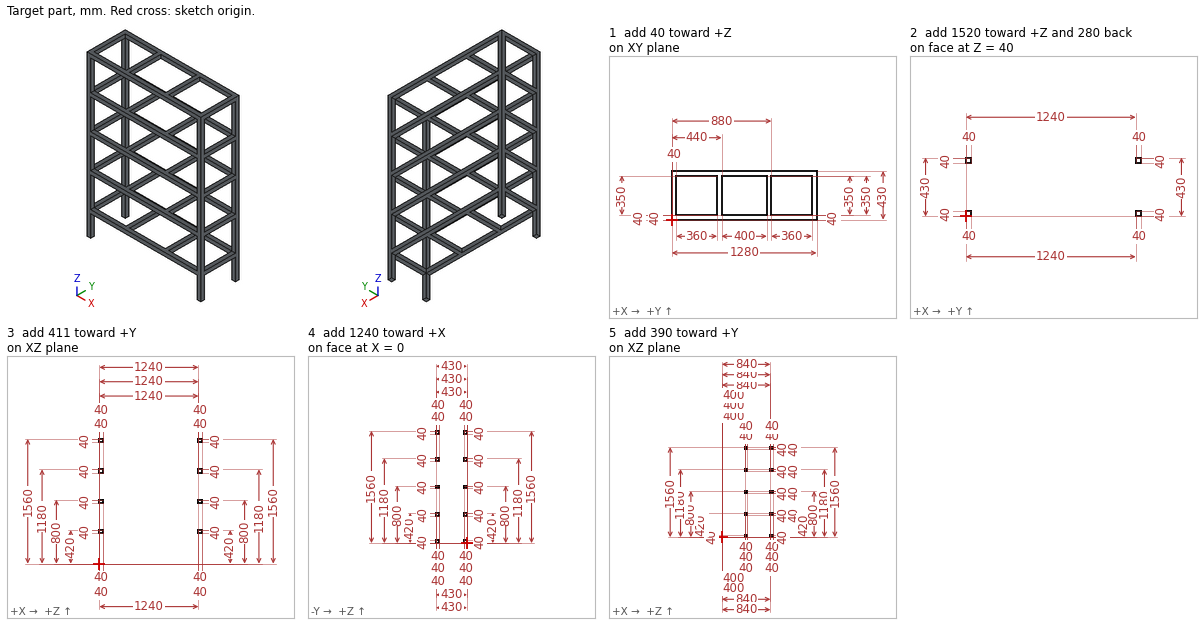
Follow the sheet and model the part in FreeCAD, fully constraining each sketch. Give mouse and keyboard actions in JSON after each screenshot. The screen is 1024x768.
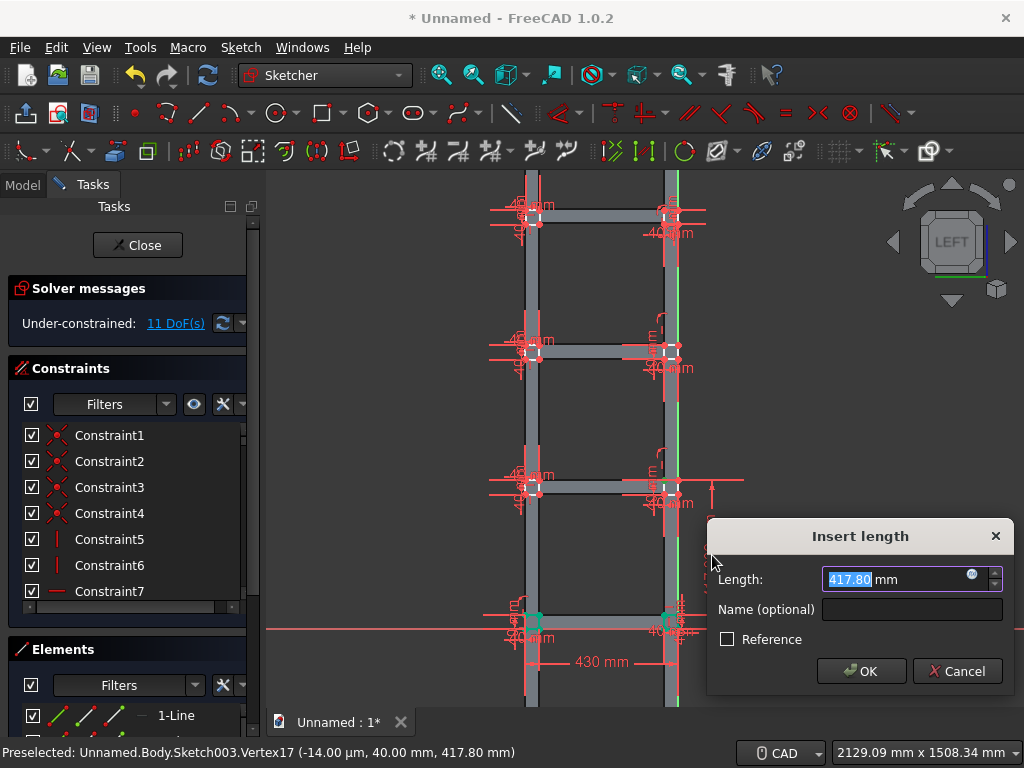
{"action": "type", "text": "420"}
{"action": "key", "text": "Return"}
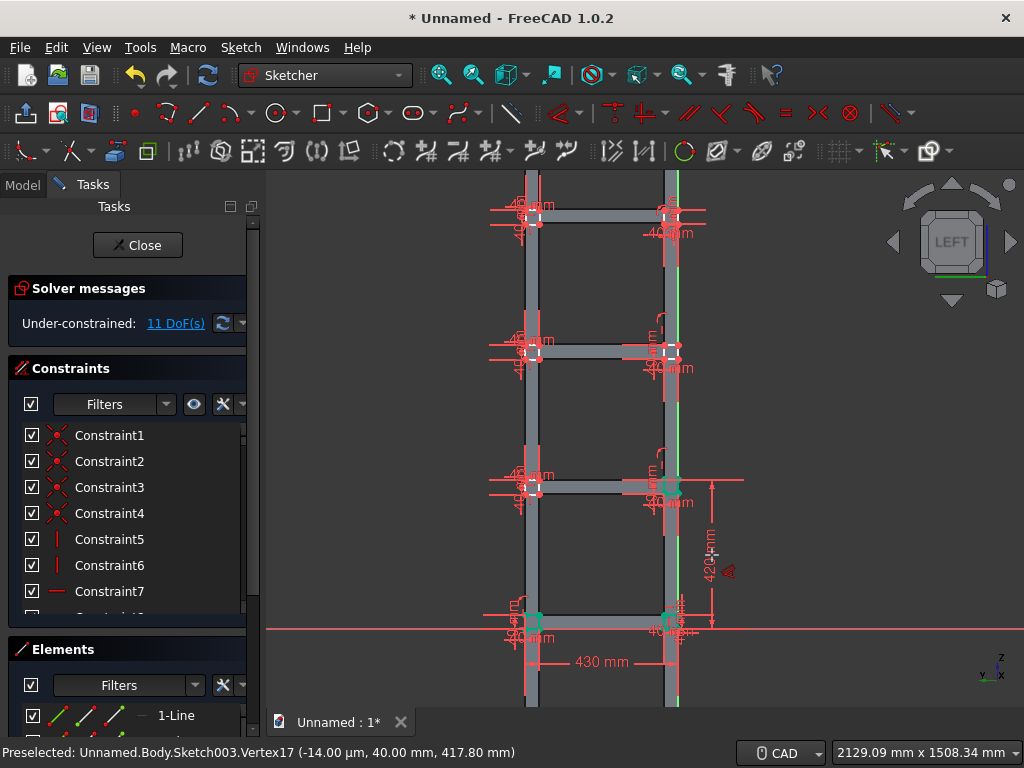
{"action": "left_click", "coordinate": [525, 480]}
{"action": "left_click", "coordinate": [602, 446]}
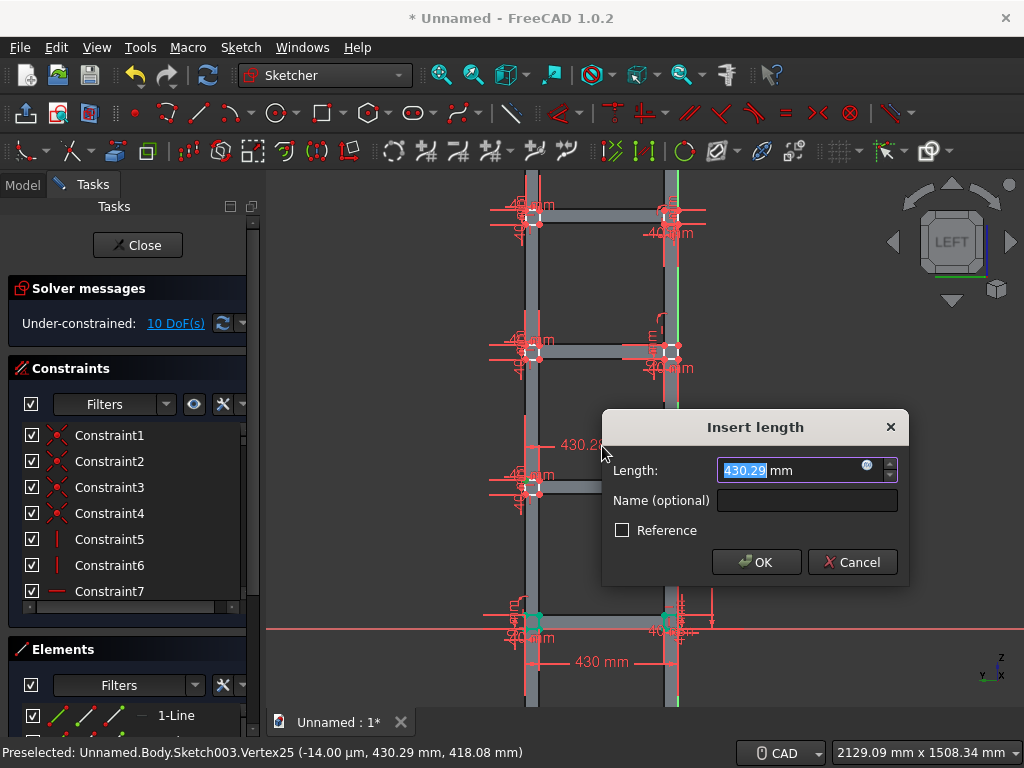
{"action": "type", "text": "430"}
{"action": "key", "text": "Return"}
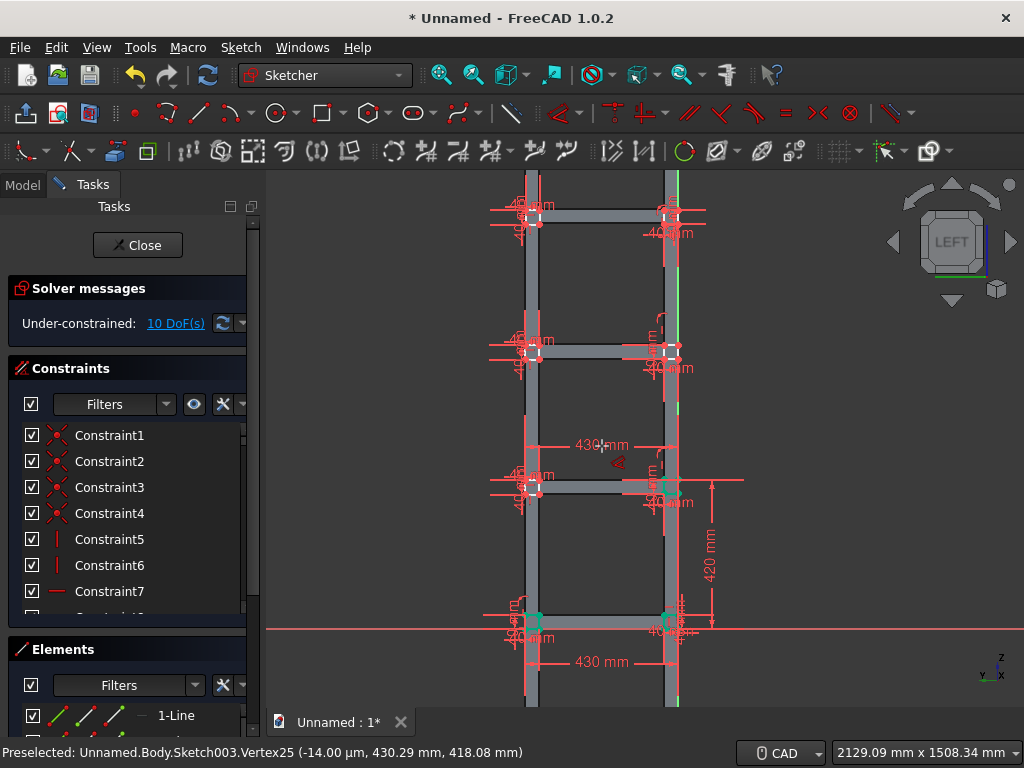
{"action": "left_click", "coordinate": [525, 480]}
{"action": "left_click", "coordinate": [712, 589]}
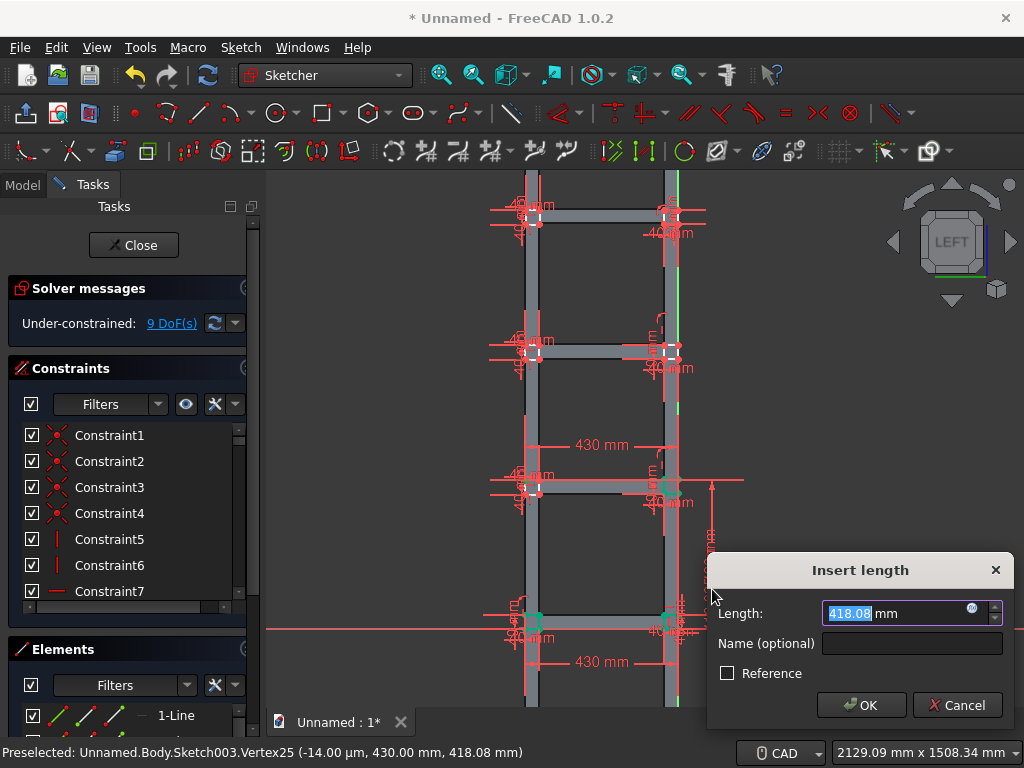
{"action": "type", "text": "420"}
{"action": "key", "text": "Return"}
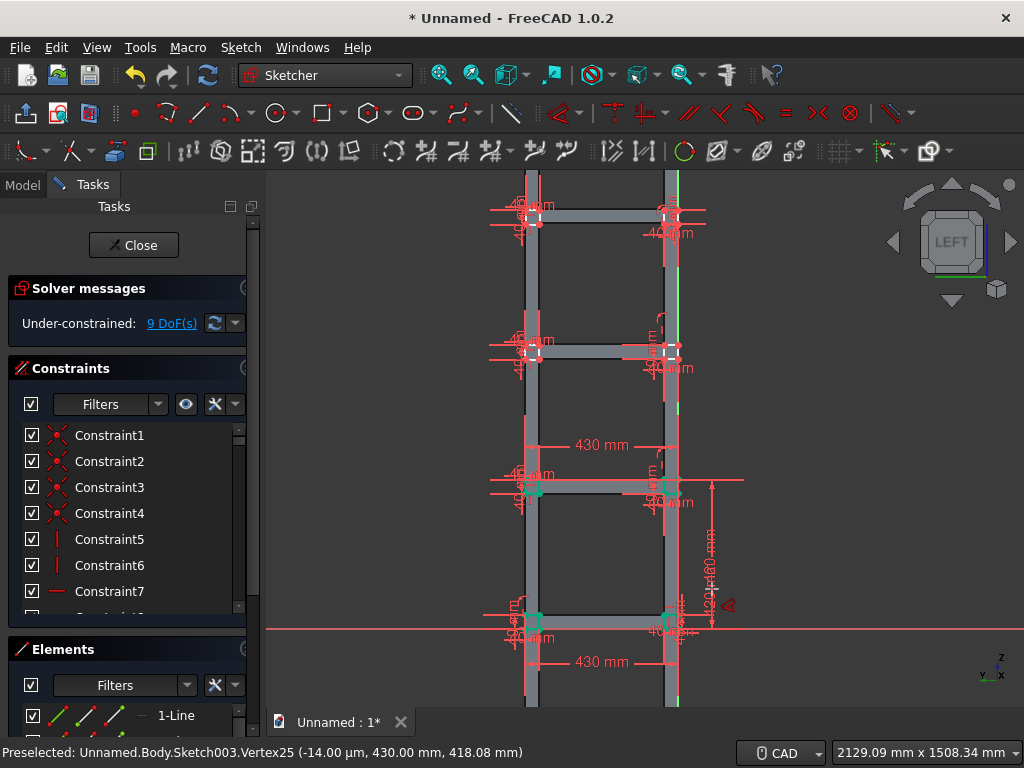
{"action": "left_click", "coordinate": [525, 345]}
{"action": "left_click", "coordinate": [602, 311]}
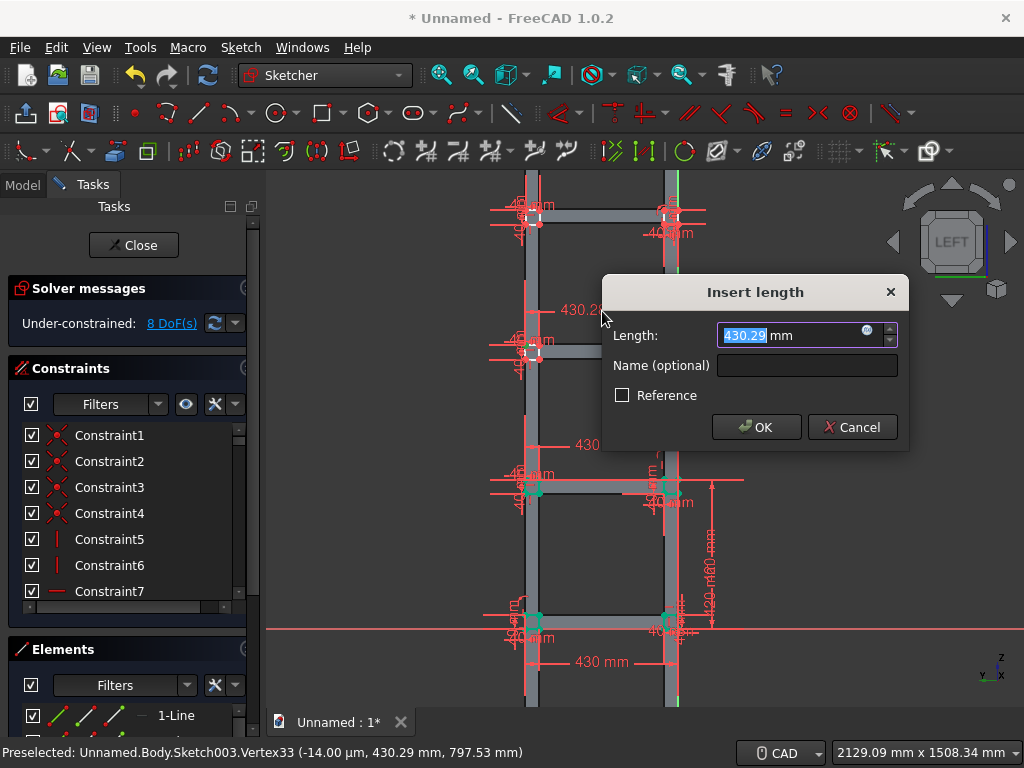
{"action": "type", "text": "430"}
{"action": "key", "text": "Return"}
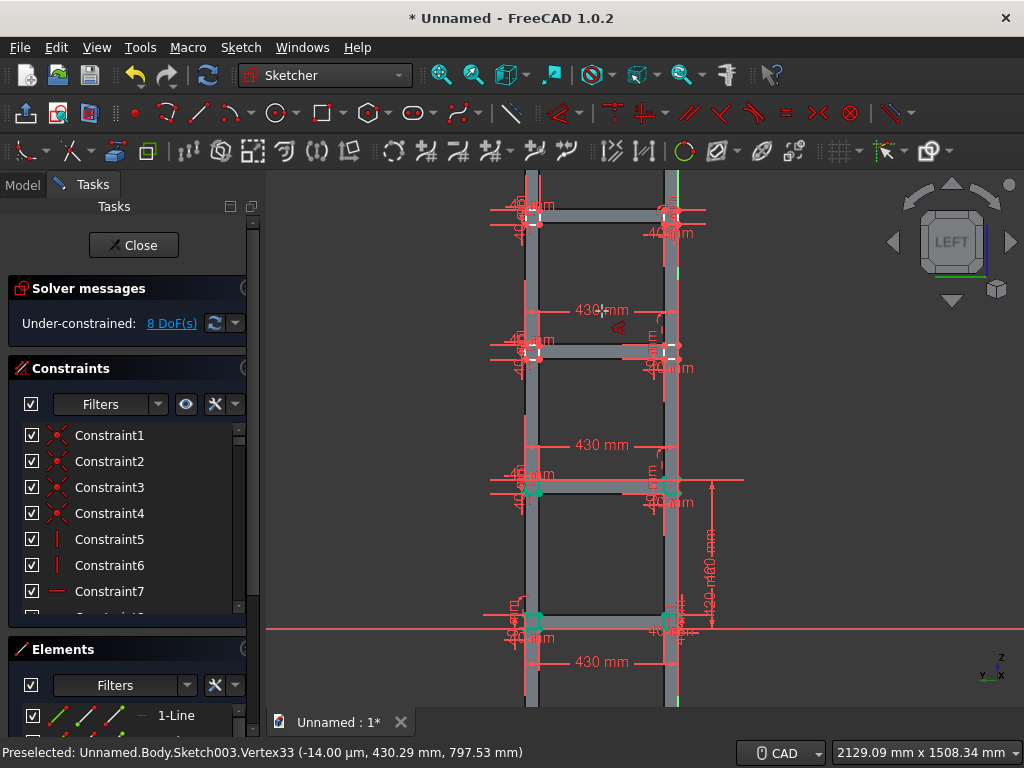
{"action": "left_click", "coordinate": [525, 345]}
{"action": "left_click", "coordinate": [712, 422]}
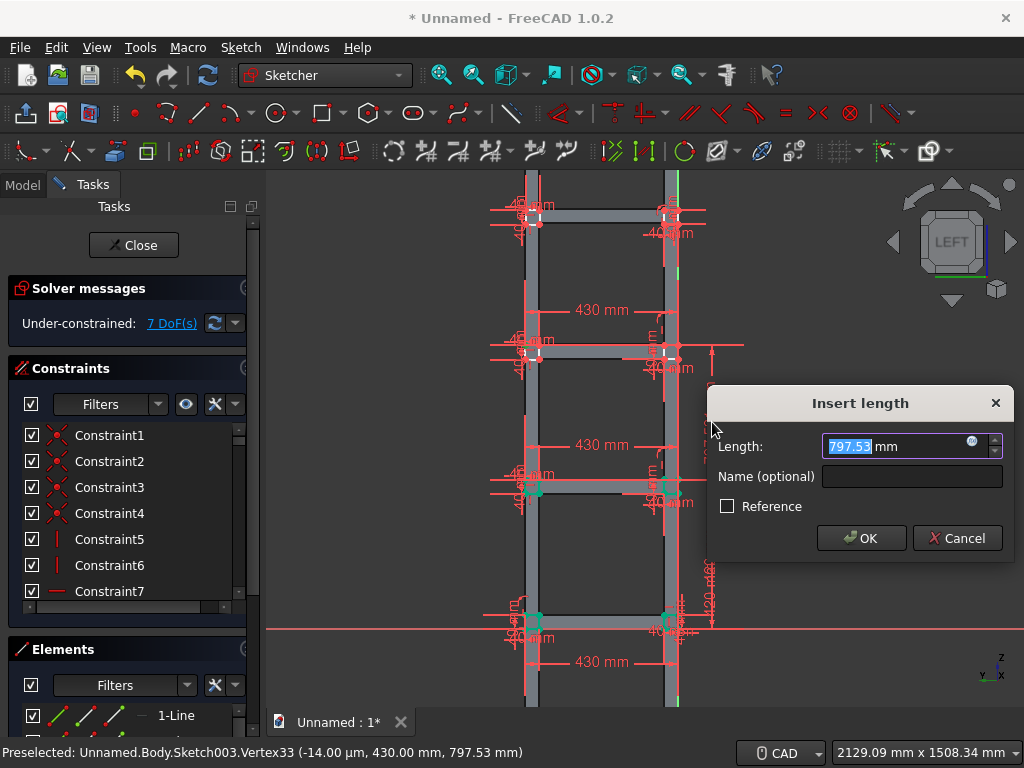
{"action": "type", "text": "800"}
{"action": "key", "text": "Return"}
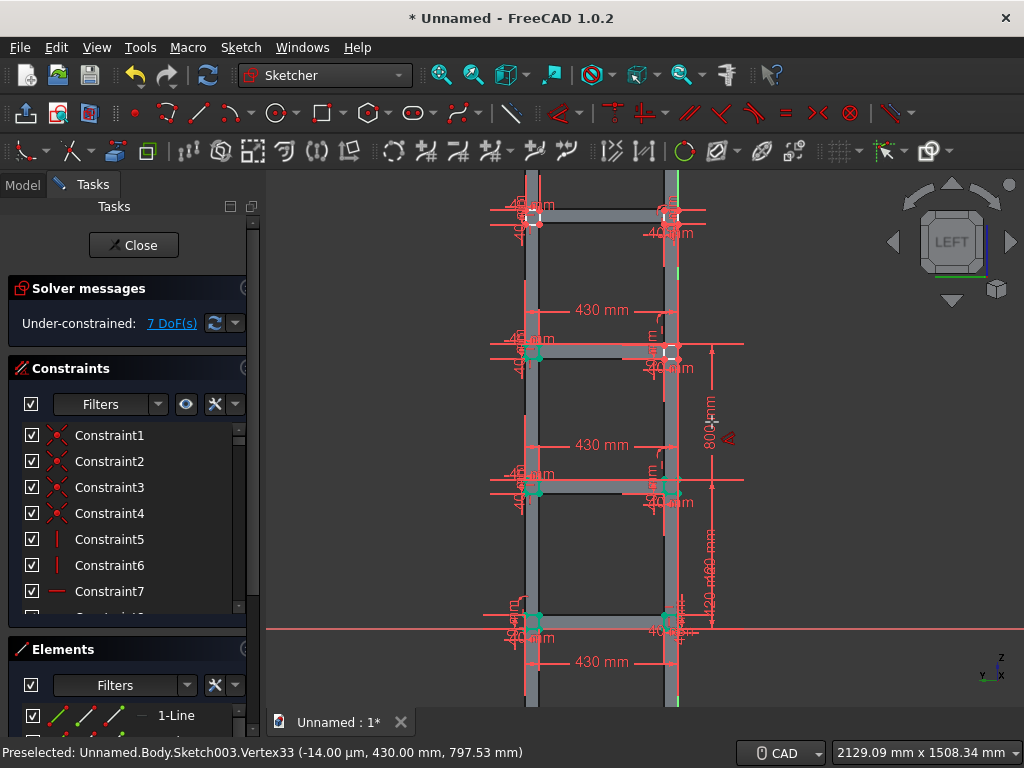
{"action": "left_click", "coordinate": [664, 345]}
{"action": "left_click", "coordinate": [630, 422]}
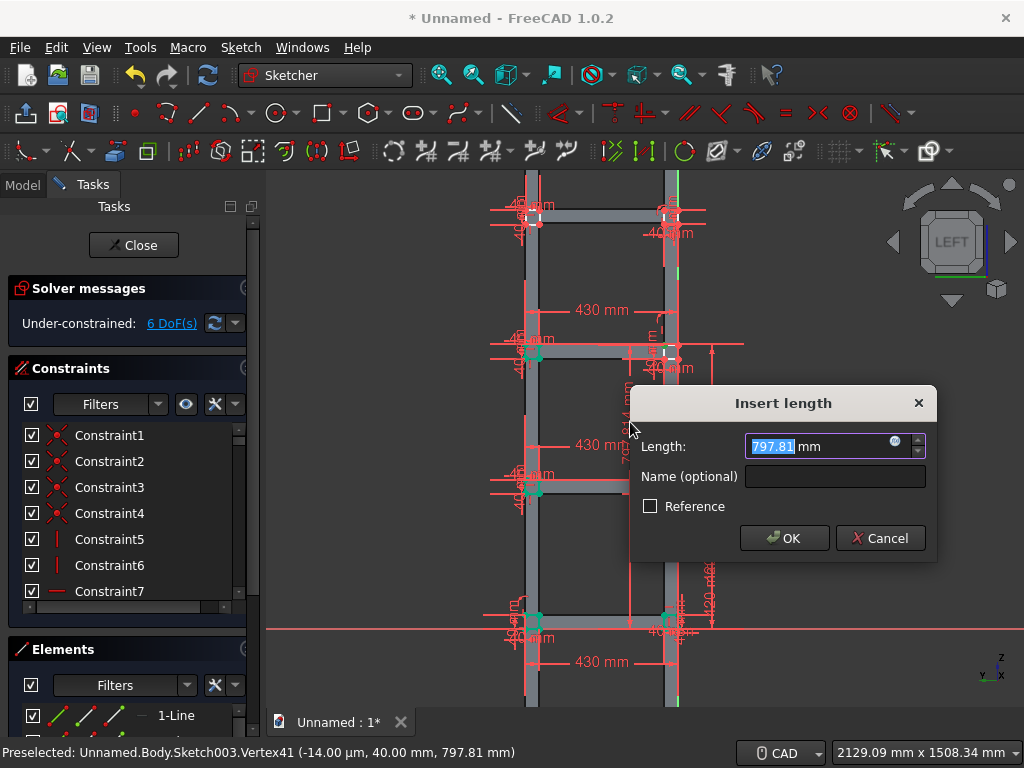
{"action": "type", "text": "800"}
{"action": "key", "text": "Return"}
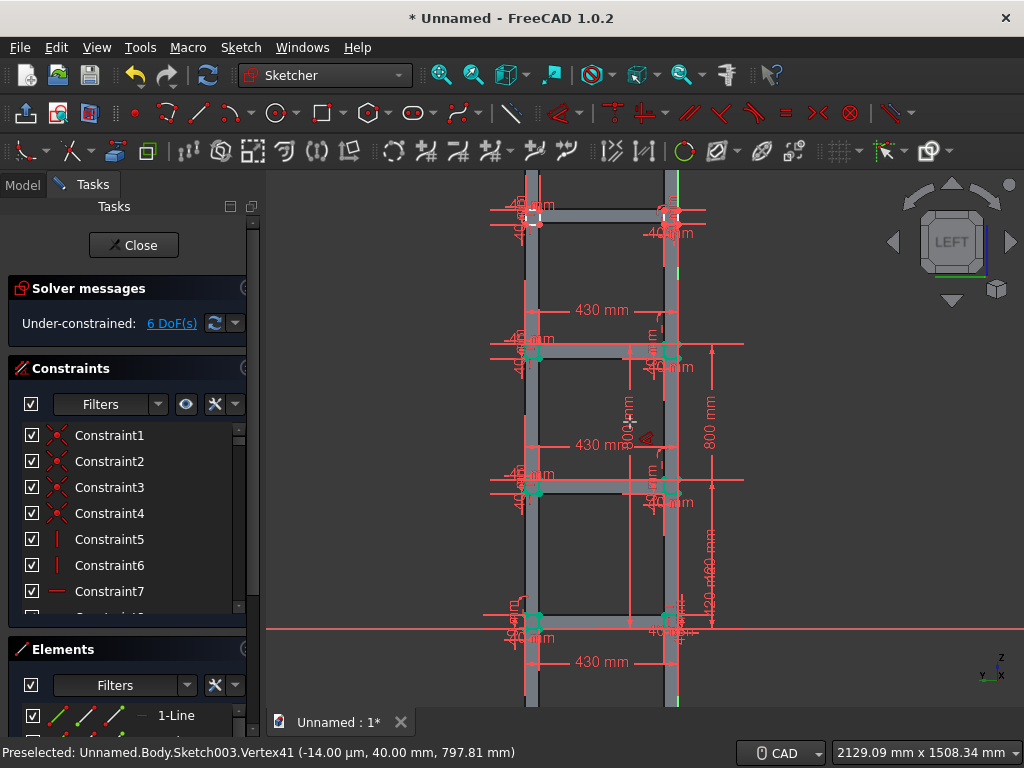
{"action": "left_click", "coordinate": [526, 210]}
{"action": "left_click", "coordinate": [637, 663]}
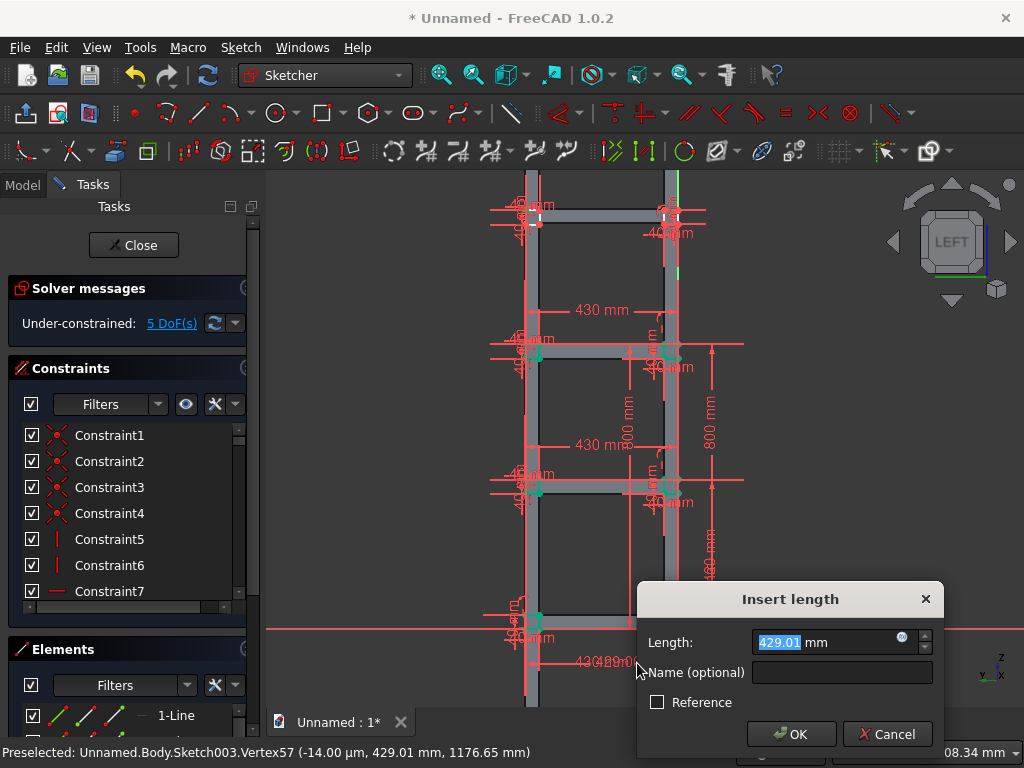
{"action": "type", "text": "430"}
{"action": "key", "text": "Return"}